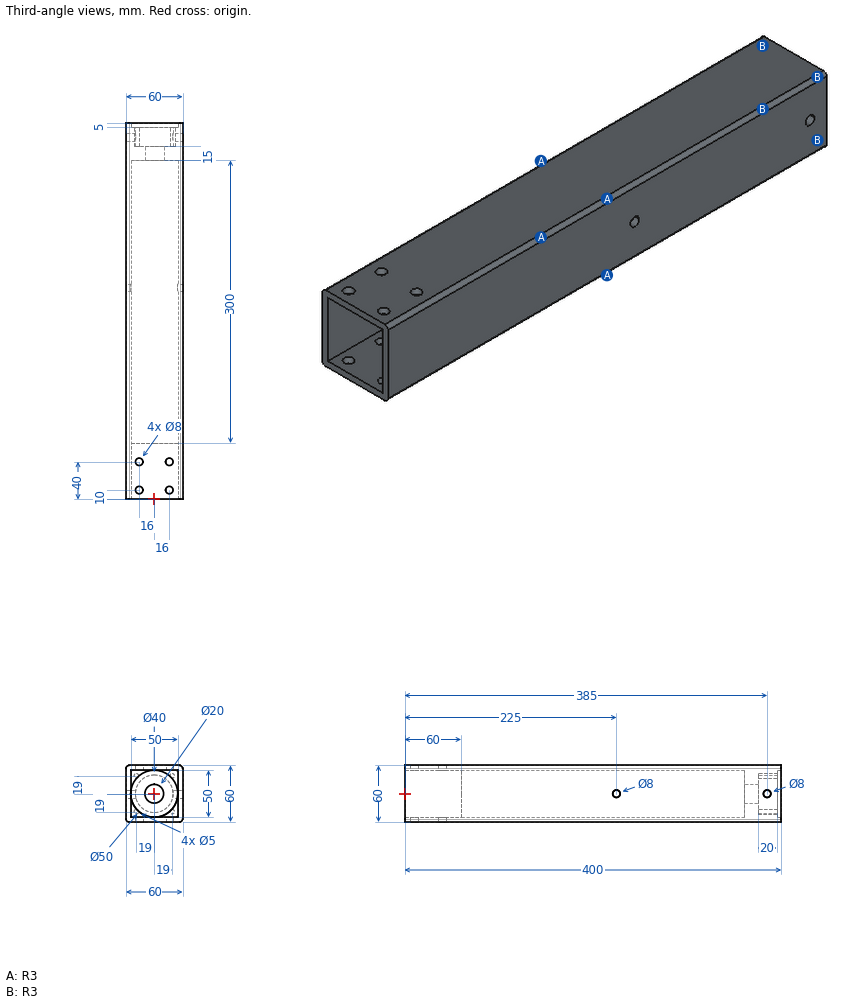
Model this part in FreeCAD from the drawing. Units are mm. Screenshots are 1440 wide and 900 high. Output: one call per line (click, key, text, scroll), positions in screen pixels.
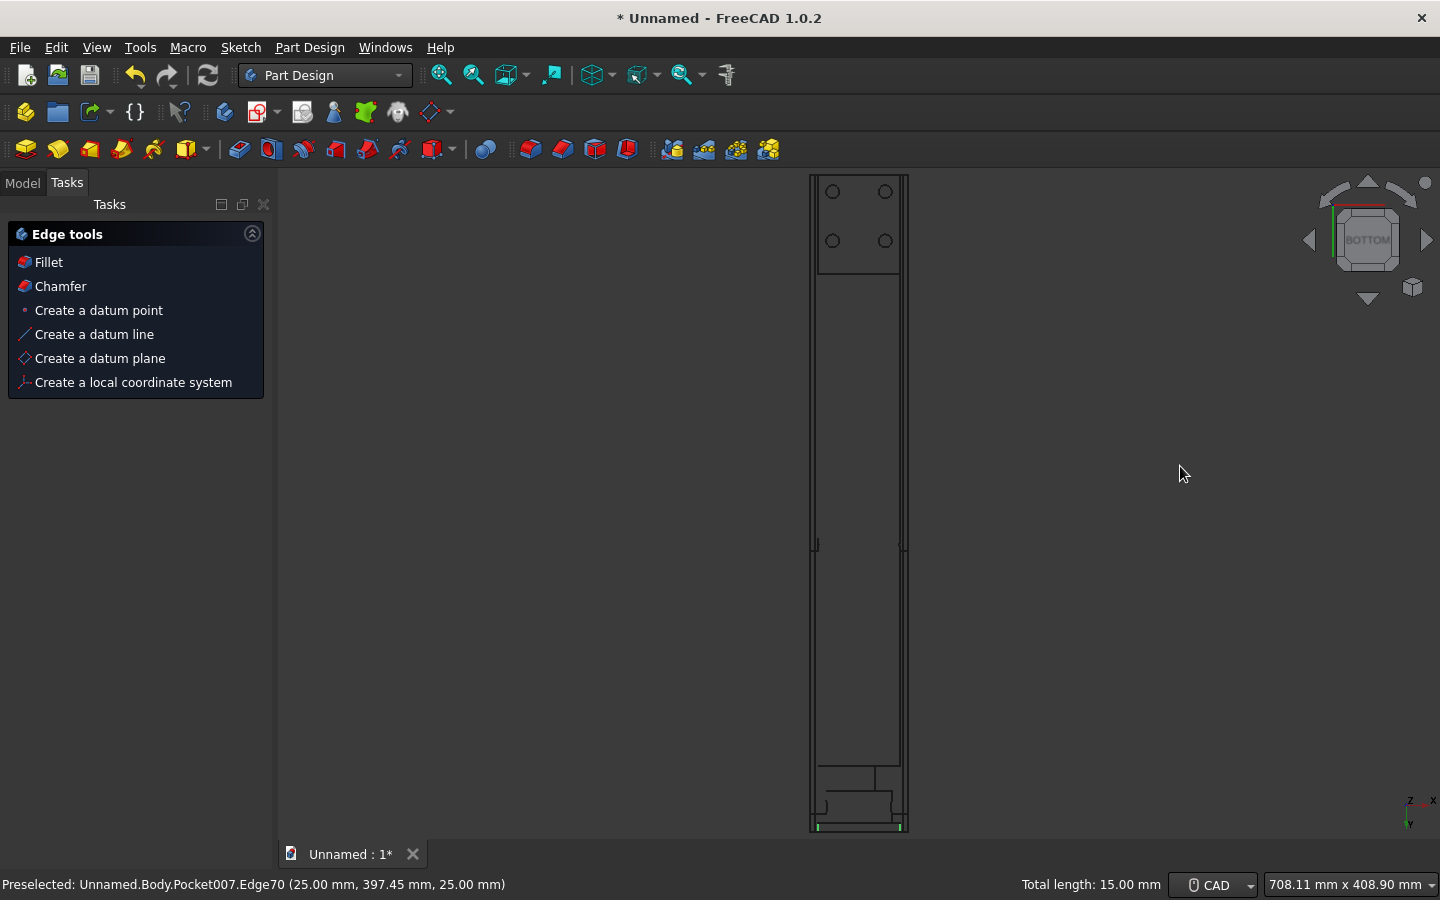
key(4)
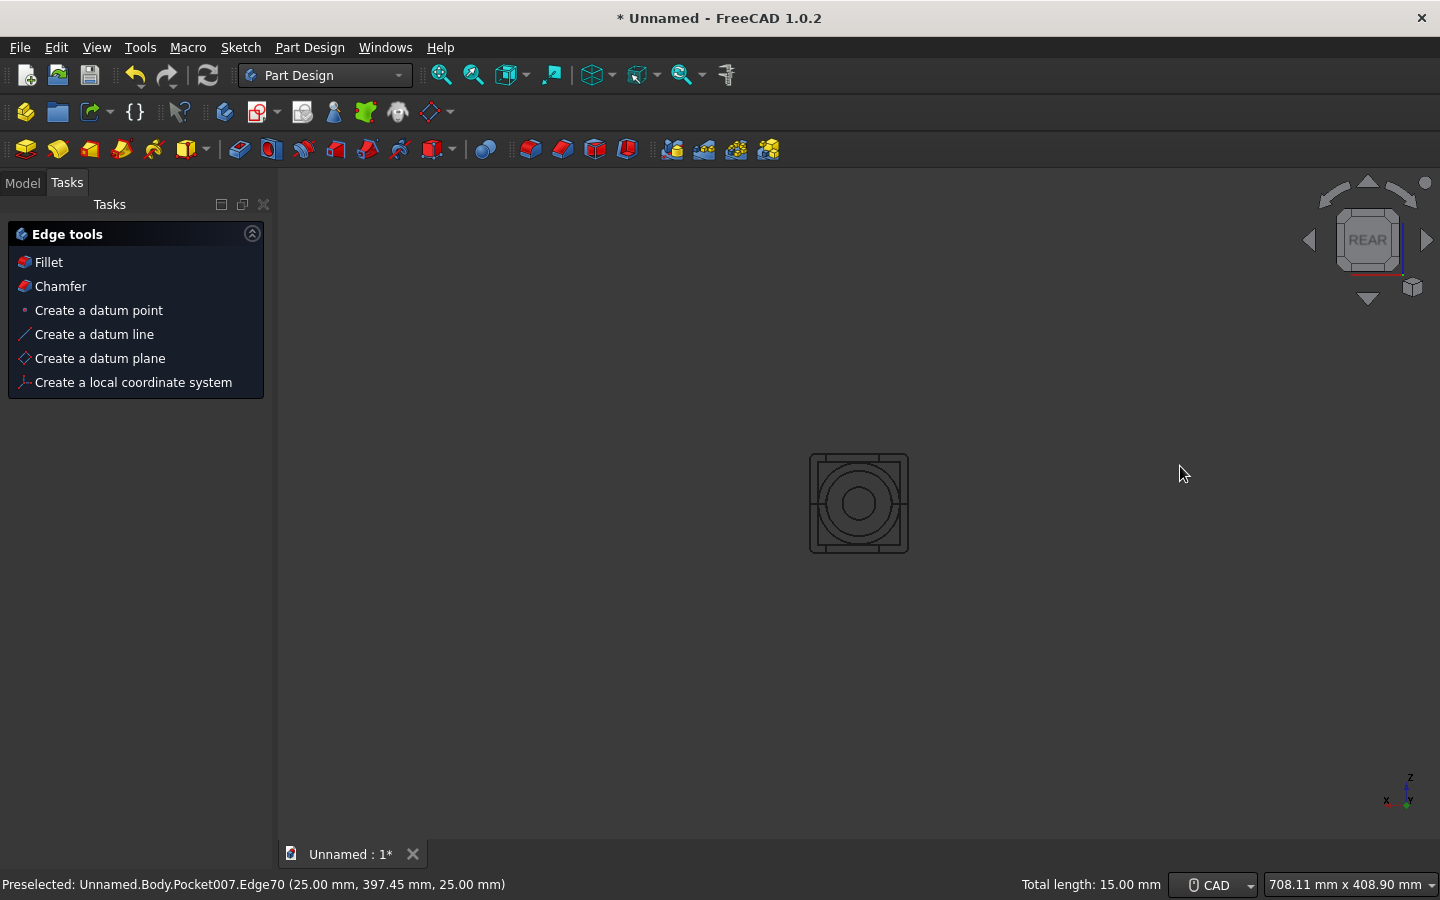
click(442, 76)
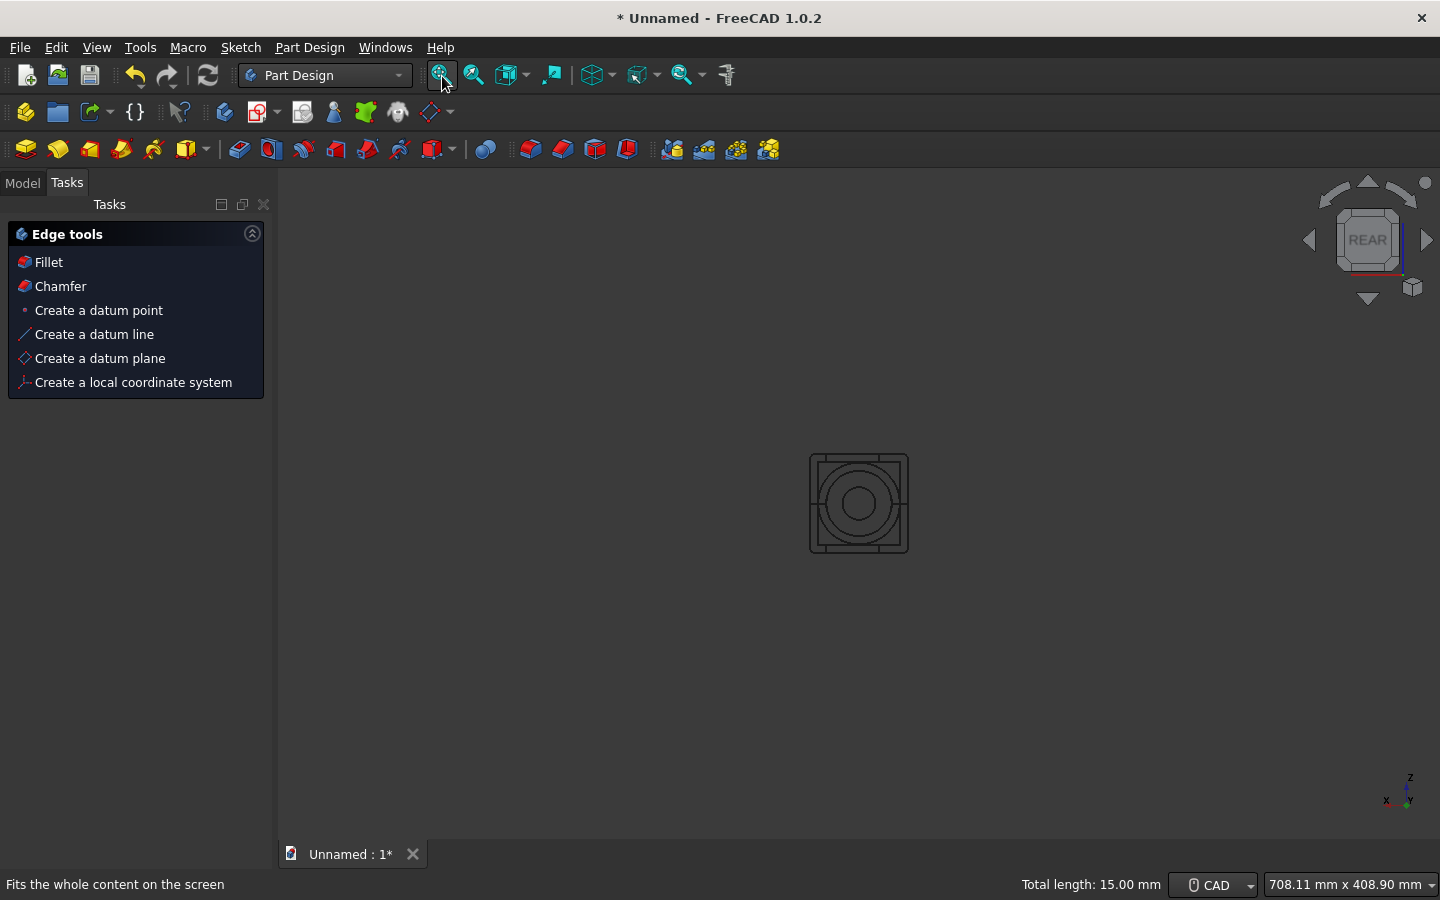
scroll(900, 461, up, 8)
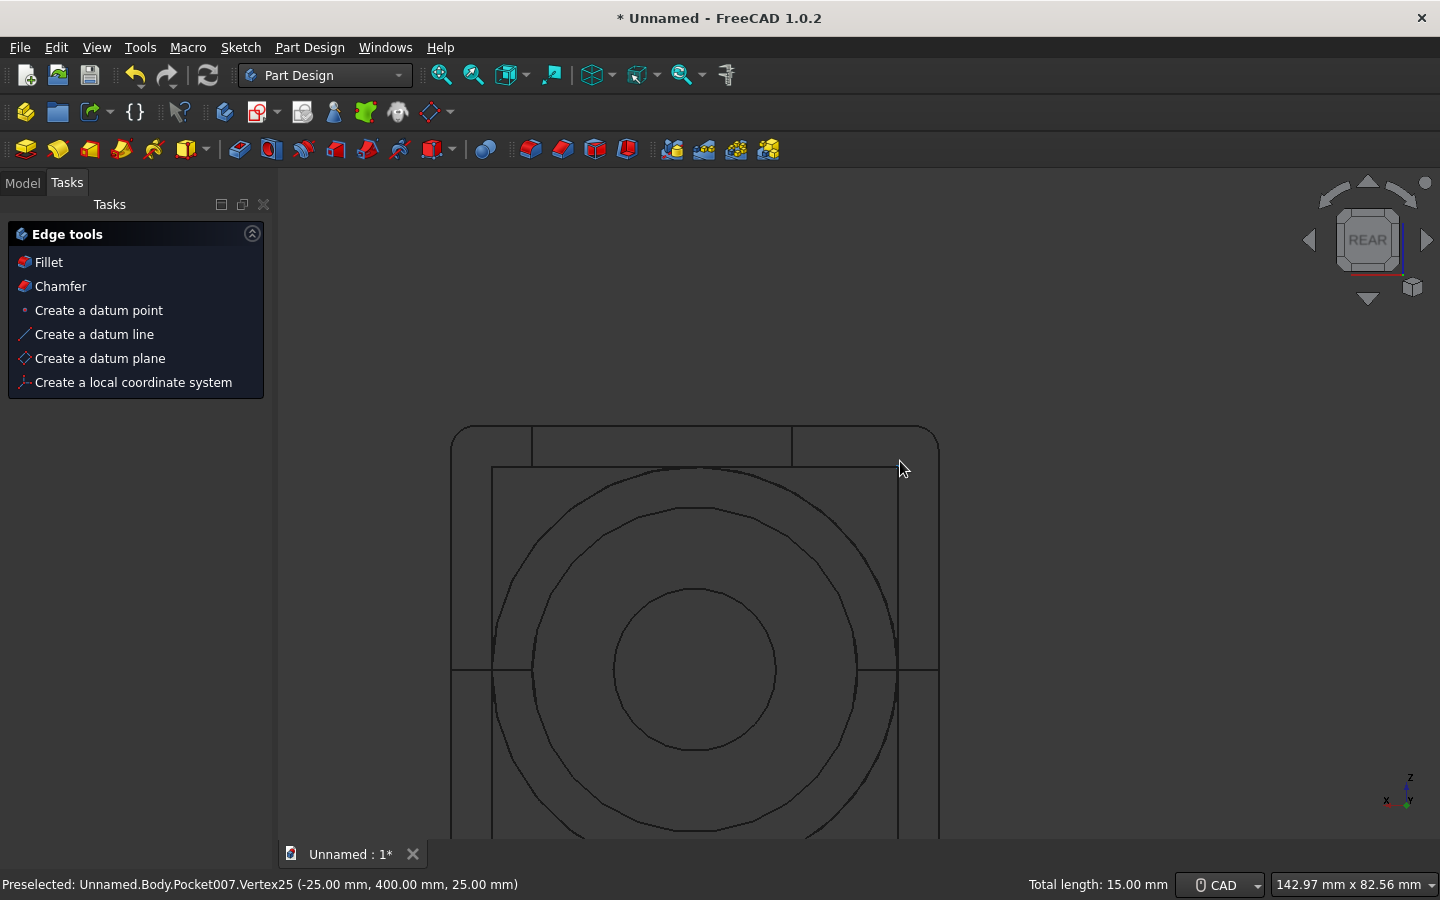
click(442, 76)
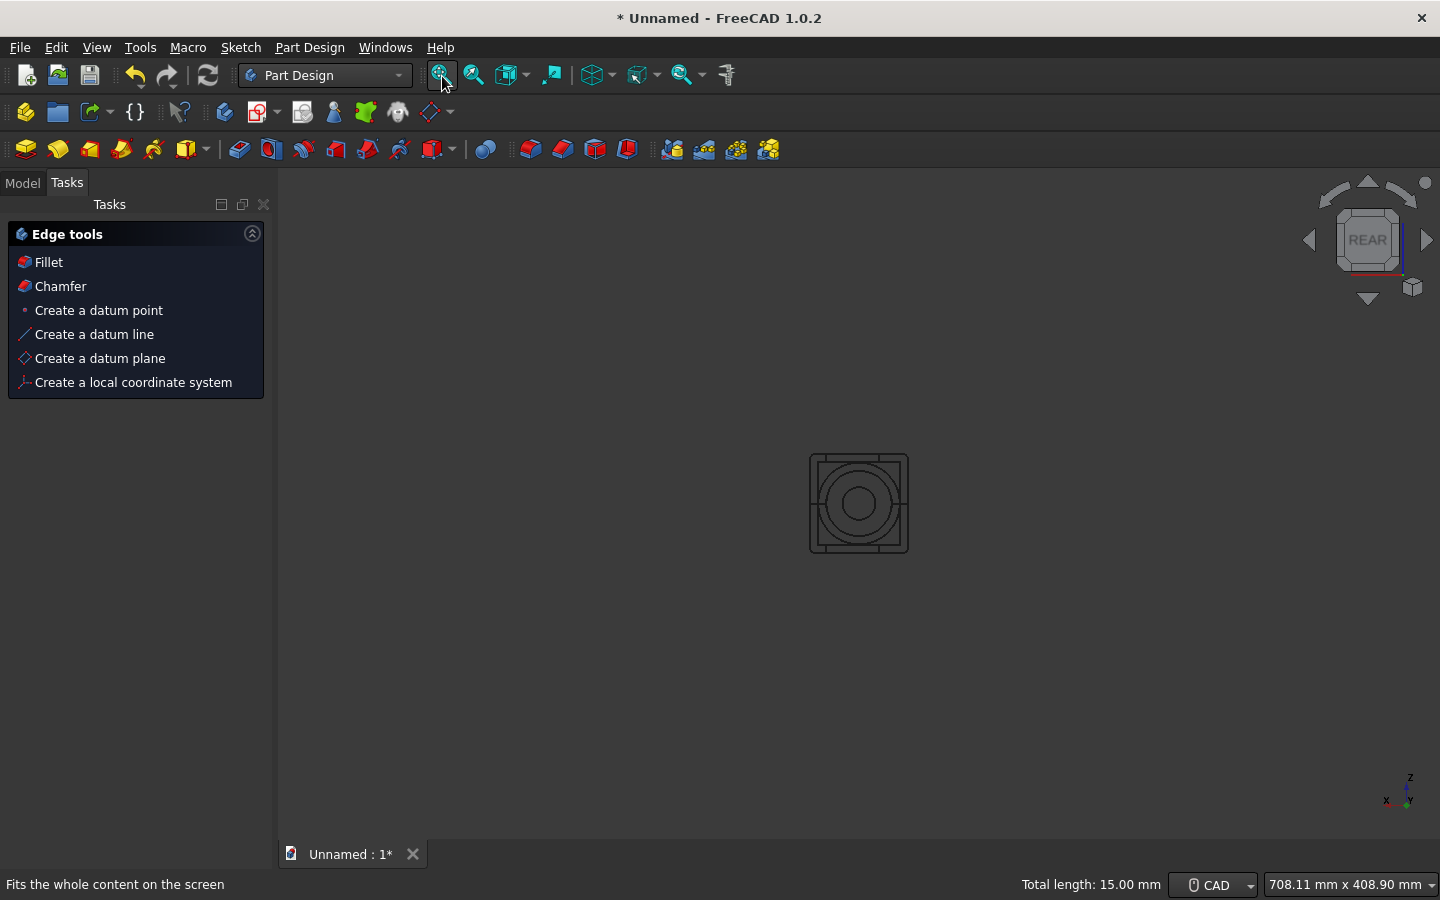
key(6)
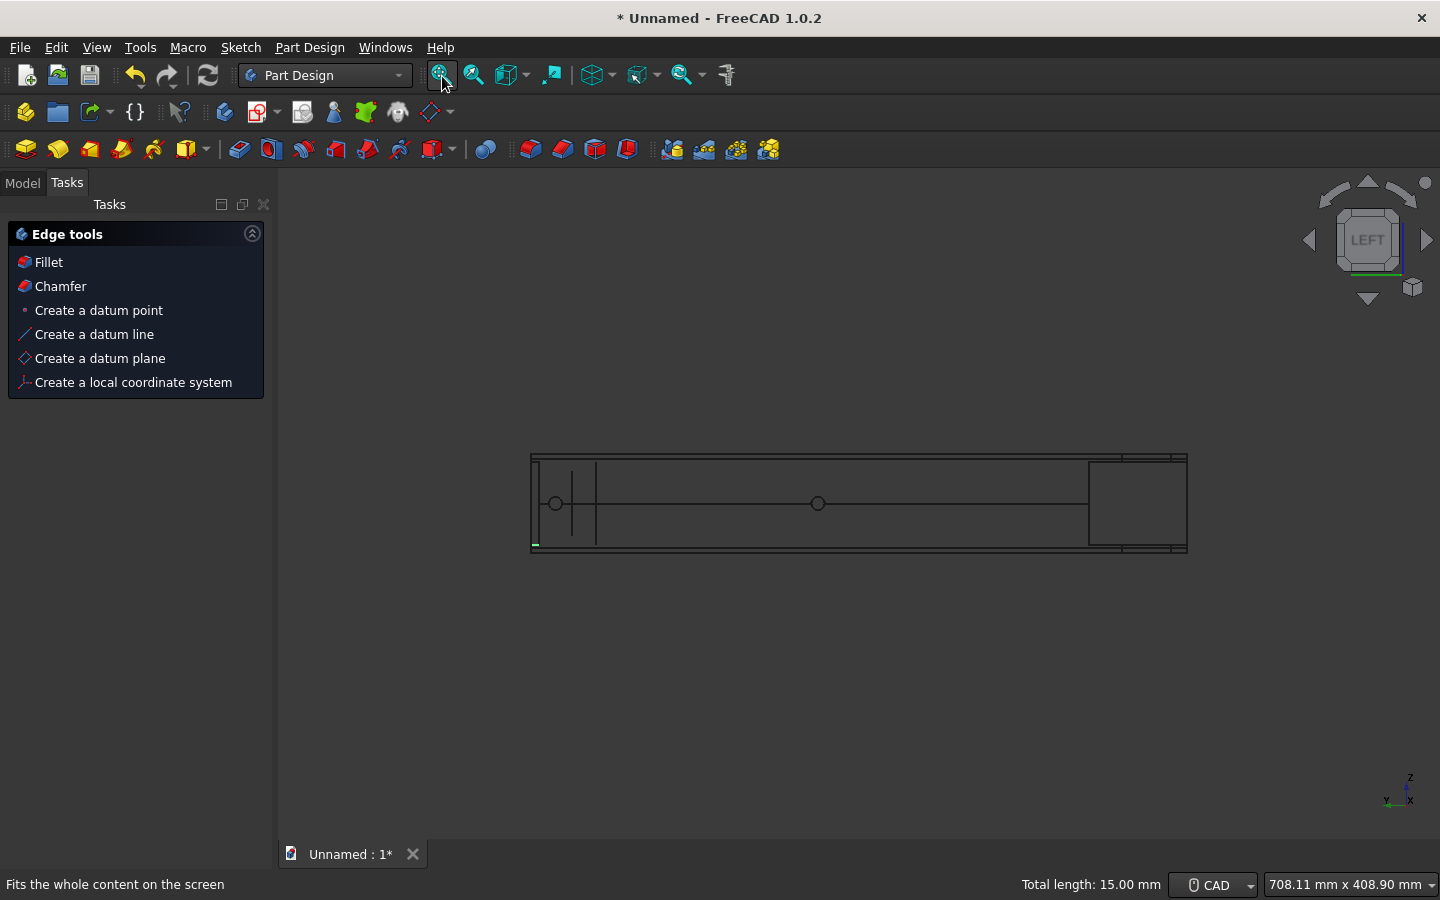
scroll(535, 461, up, 8)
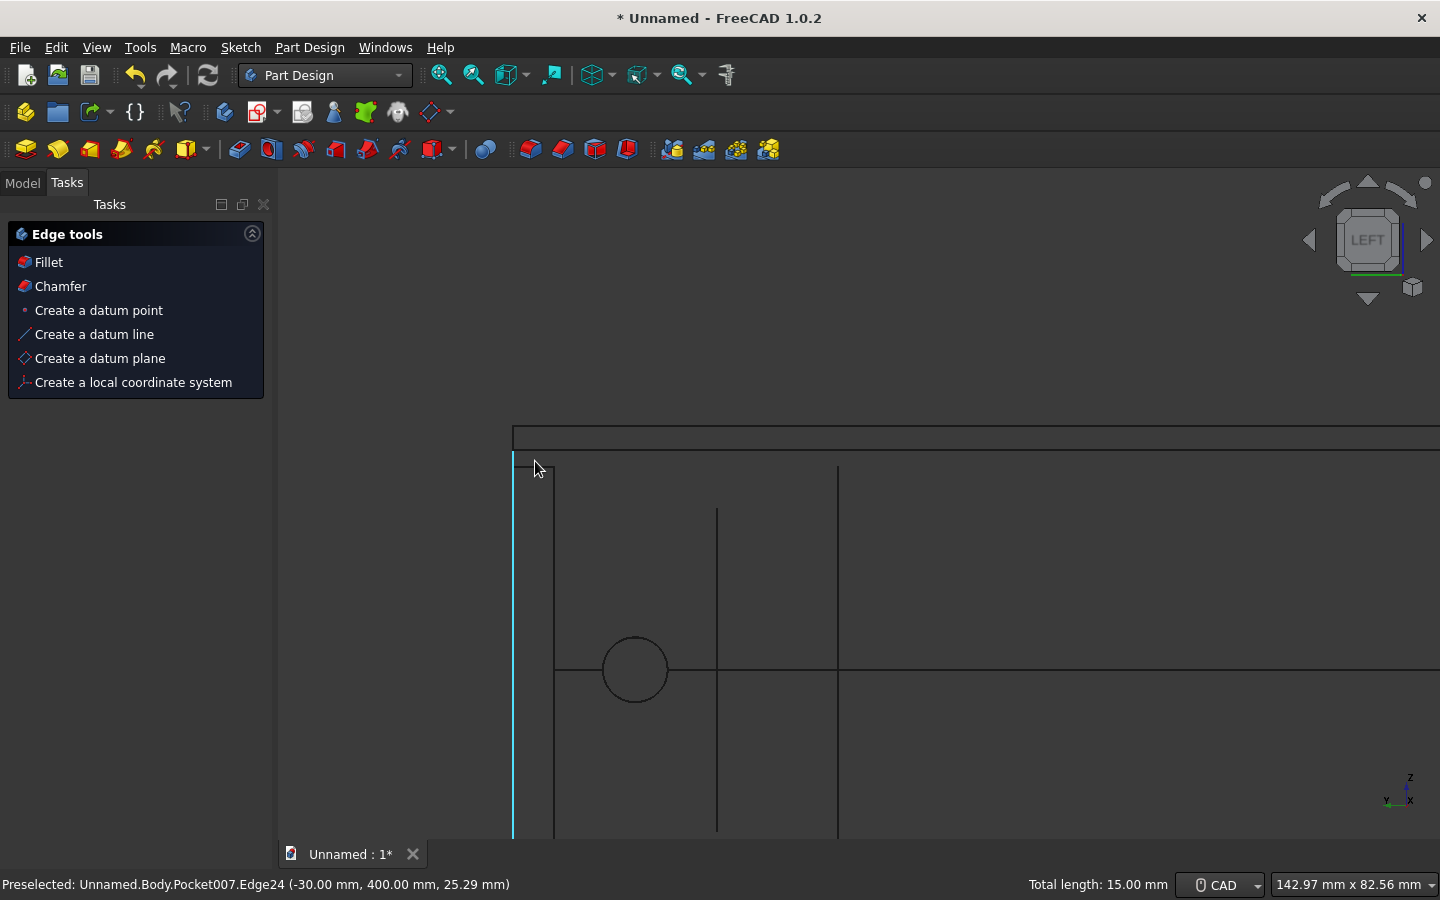
click(534, 466, ctrl)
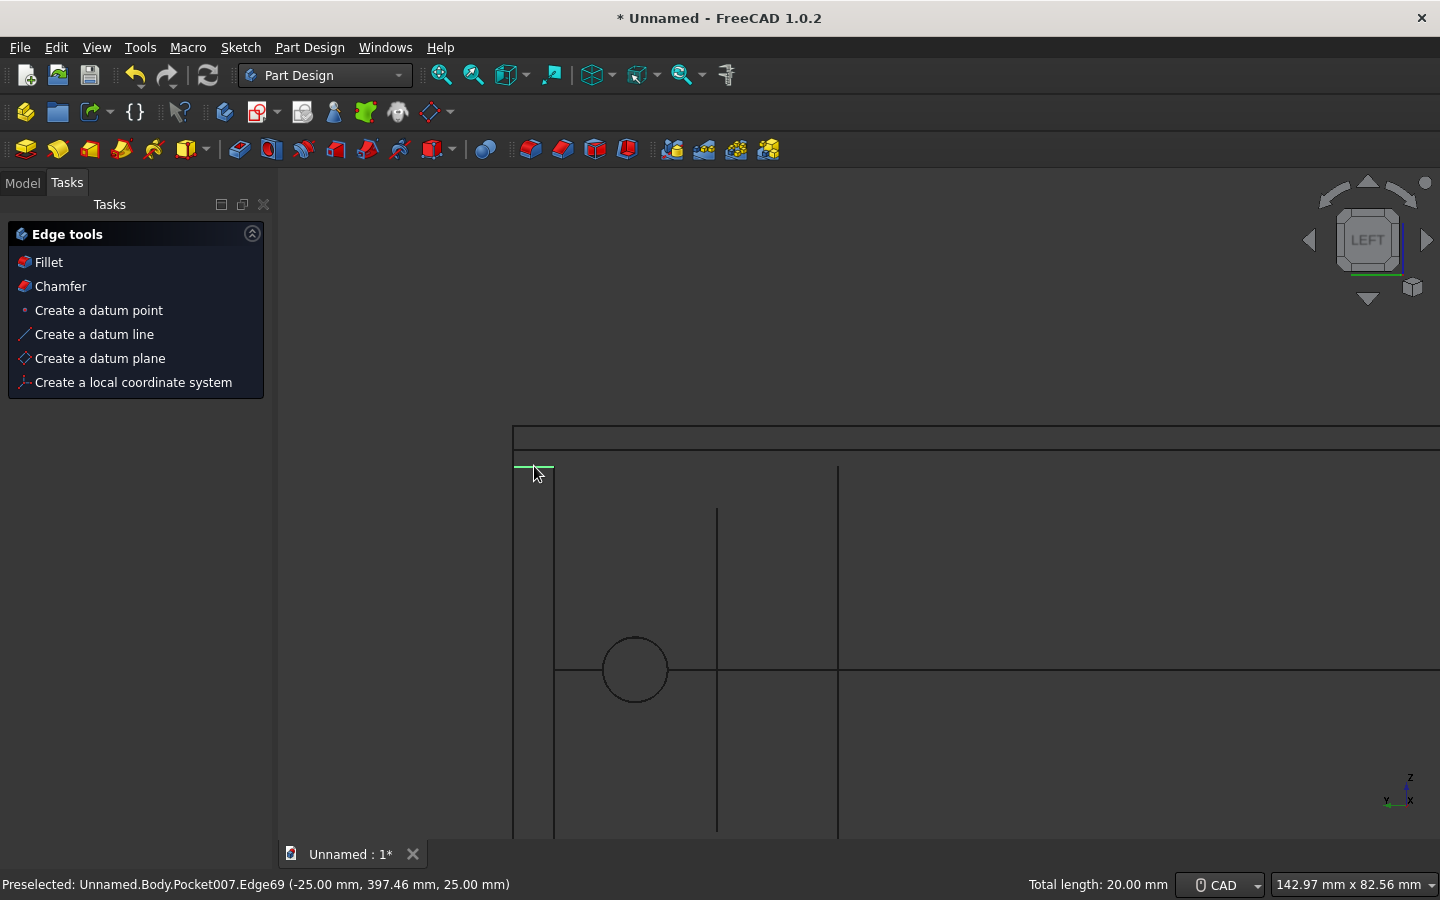
key(v)
key(1)